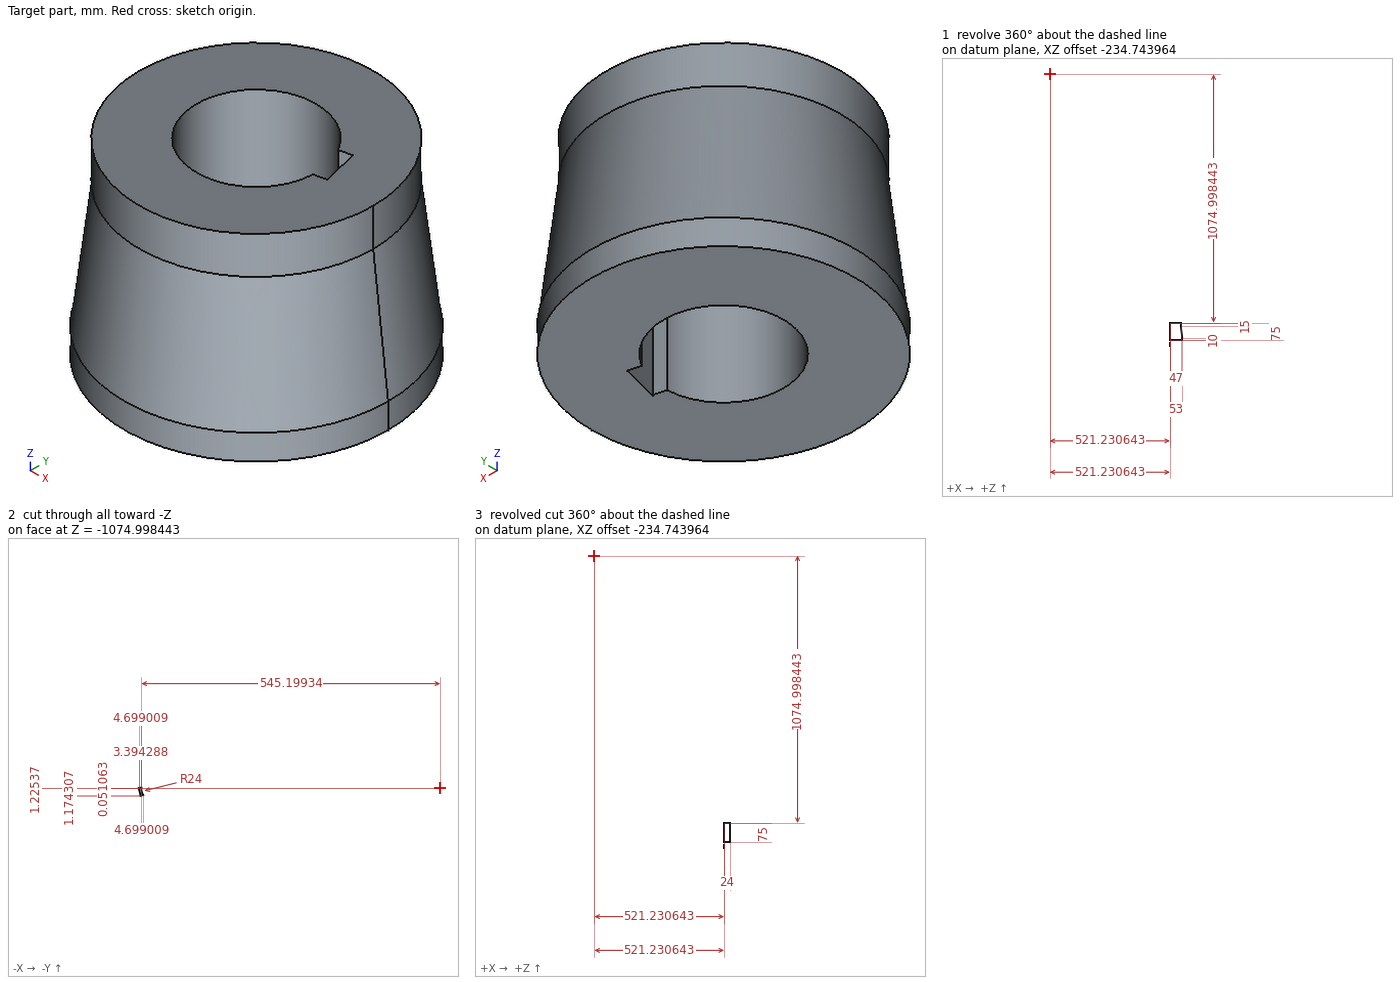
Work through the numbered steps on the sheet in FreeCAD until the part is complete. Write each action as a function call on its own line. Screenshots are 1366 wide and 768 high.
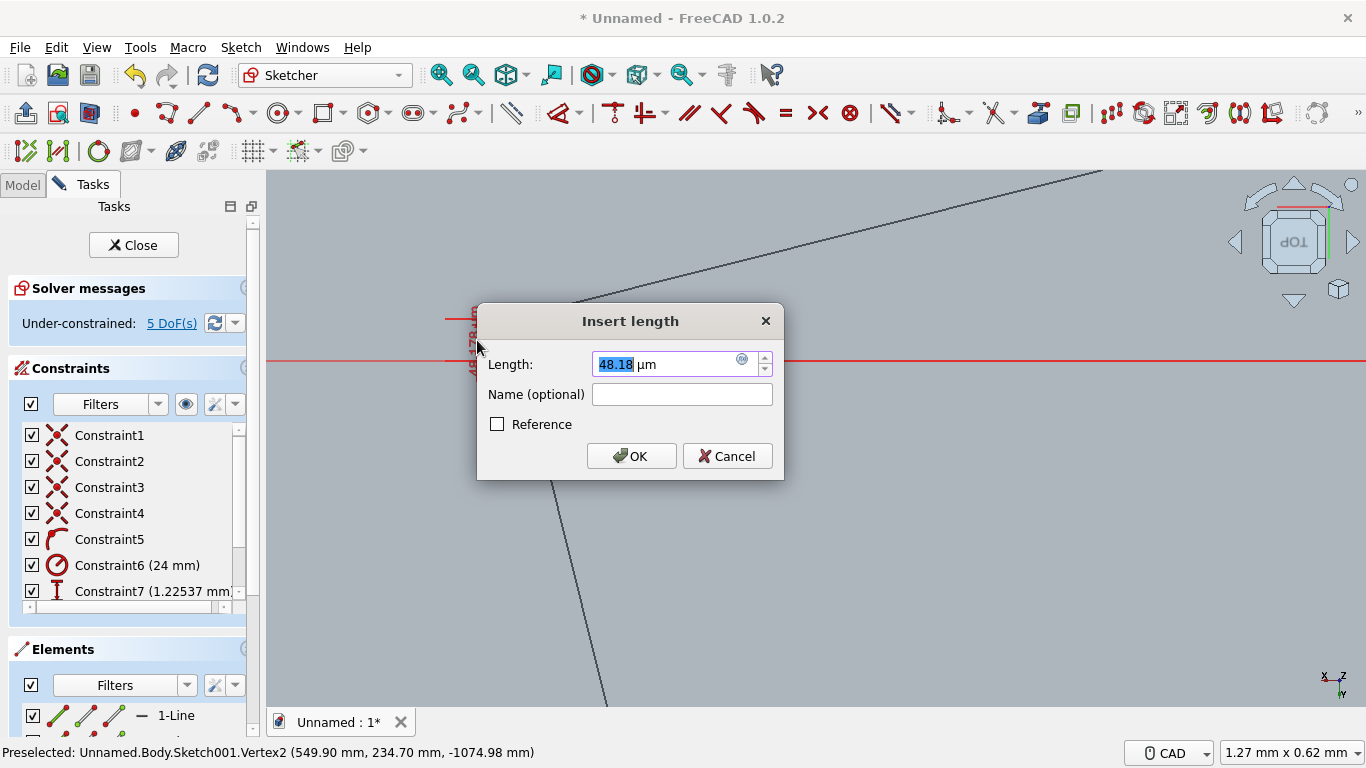
key(ctrl+a)
text(0.051063 mm)
key(Return)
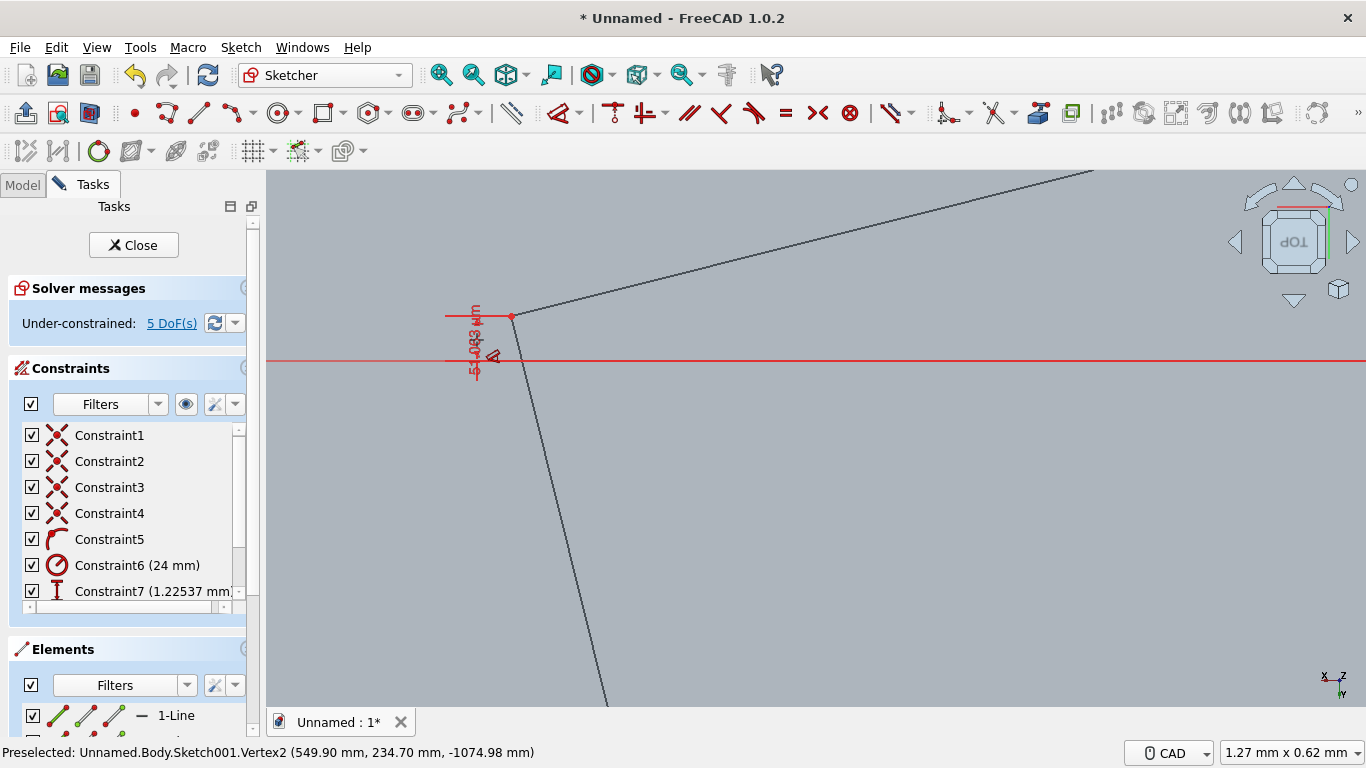
scroll(635, 257, down, 17)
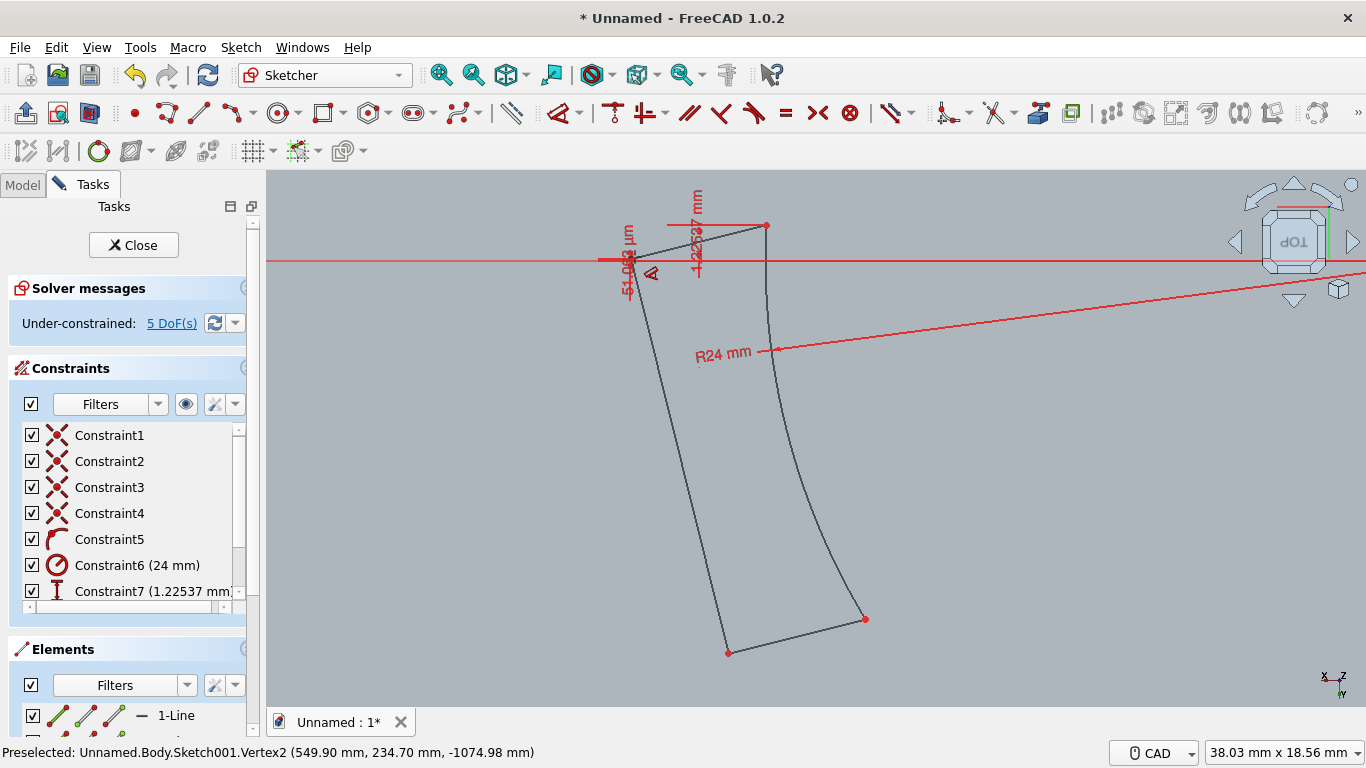
click(726, 235)
click(699, 293)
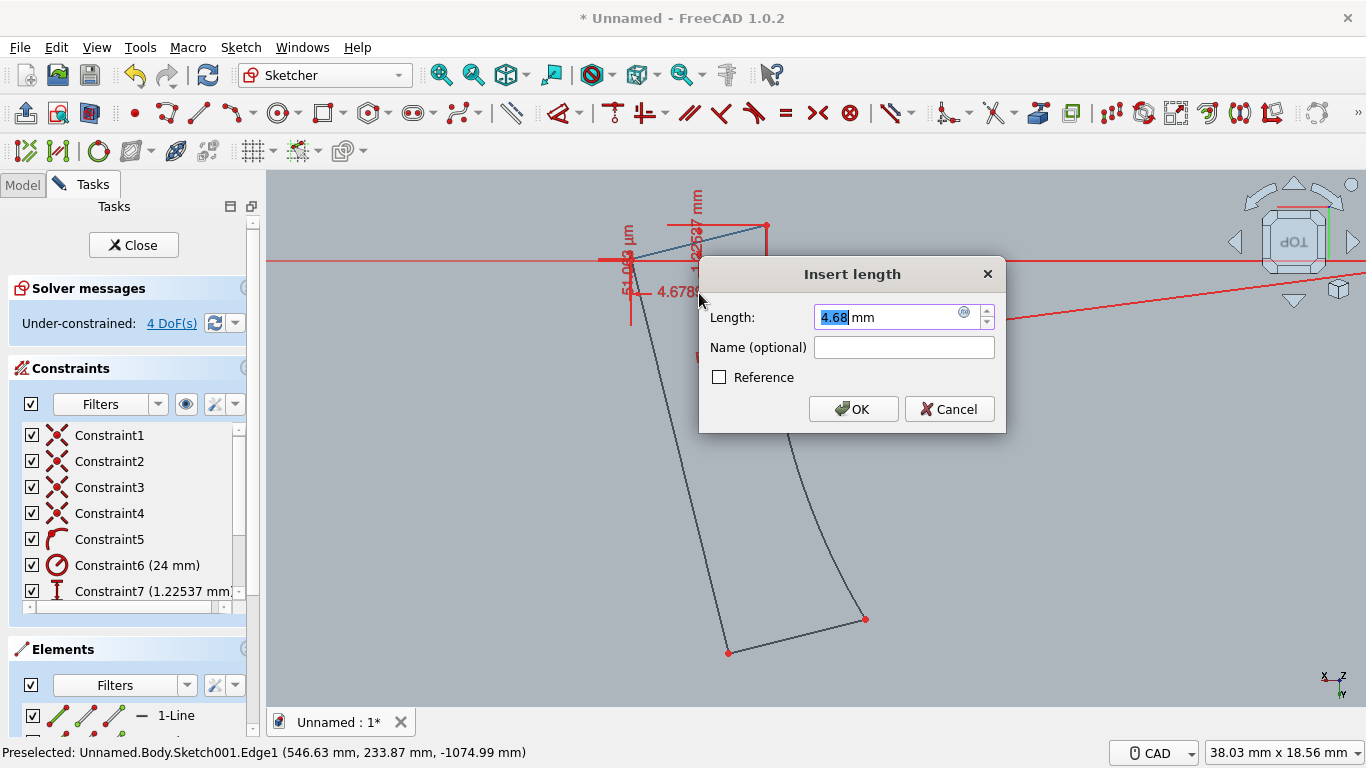
text(4.699009)
key(Return)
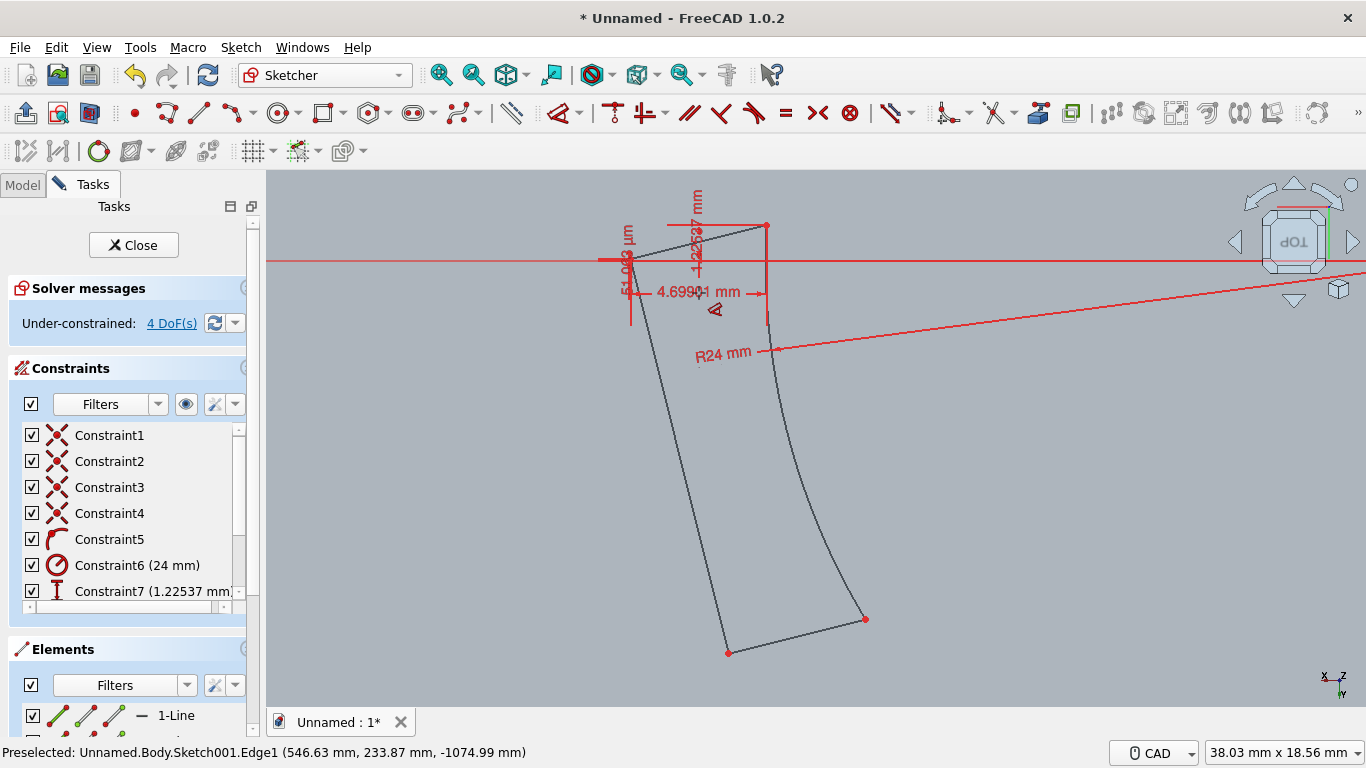
click(660, 378)
click(680, 201)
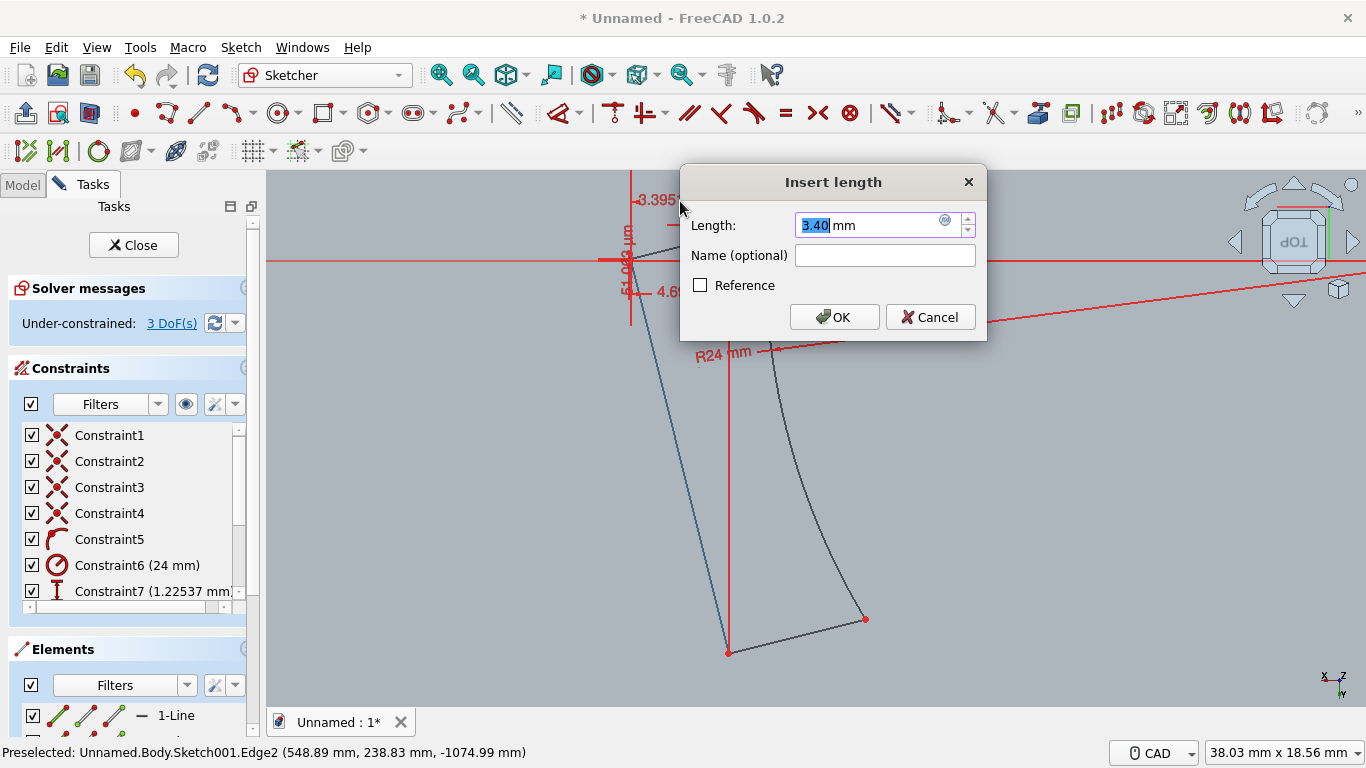
text(3.394288)
key(Return)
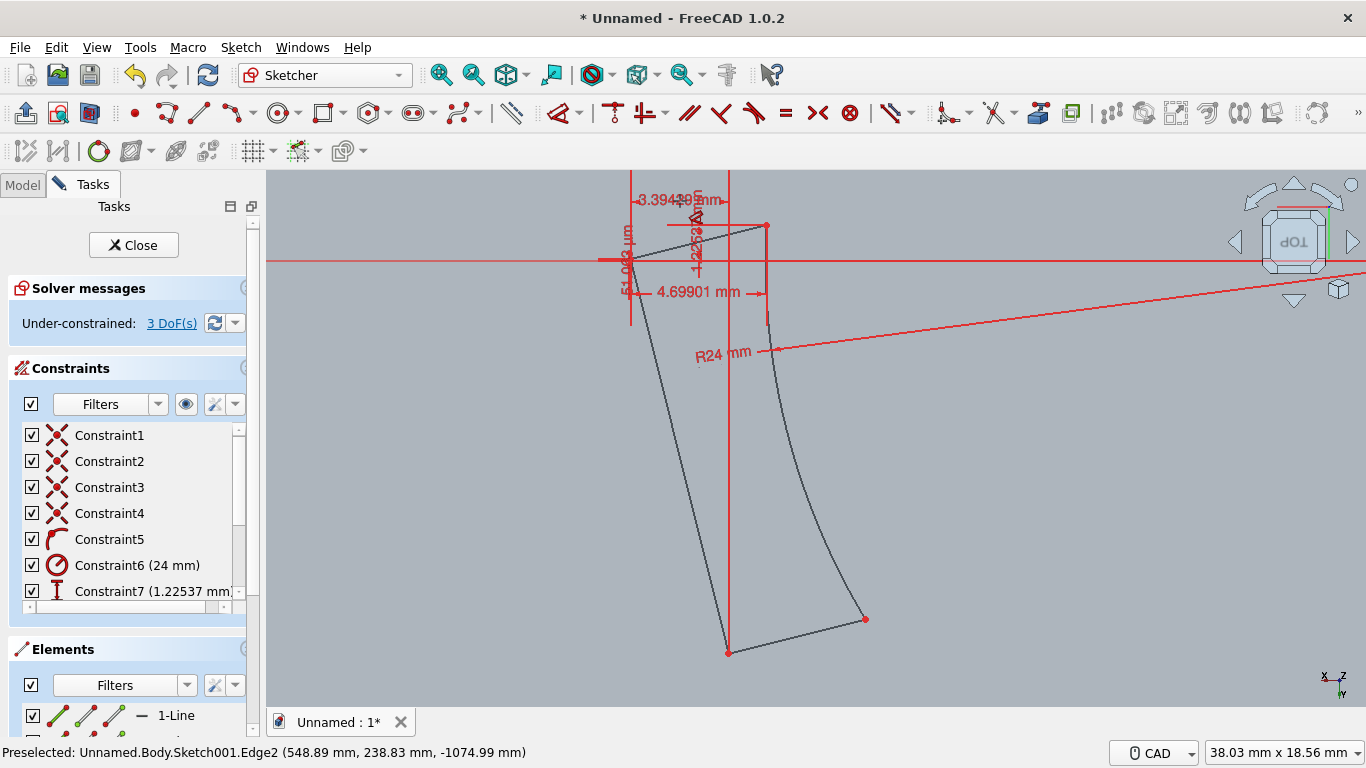
click(770, 643)
click(797, 586)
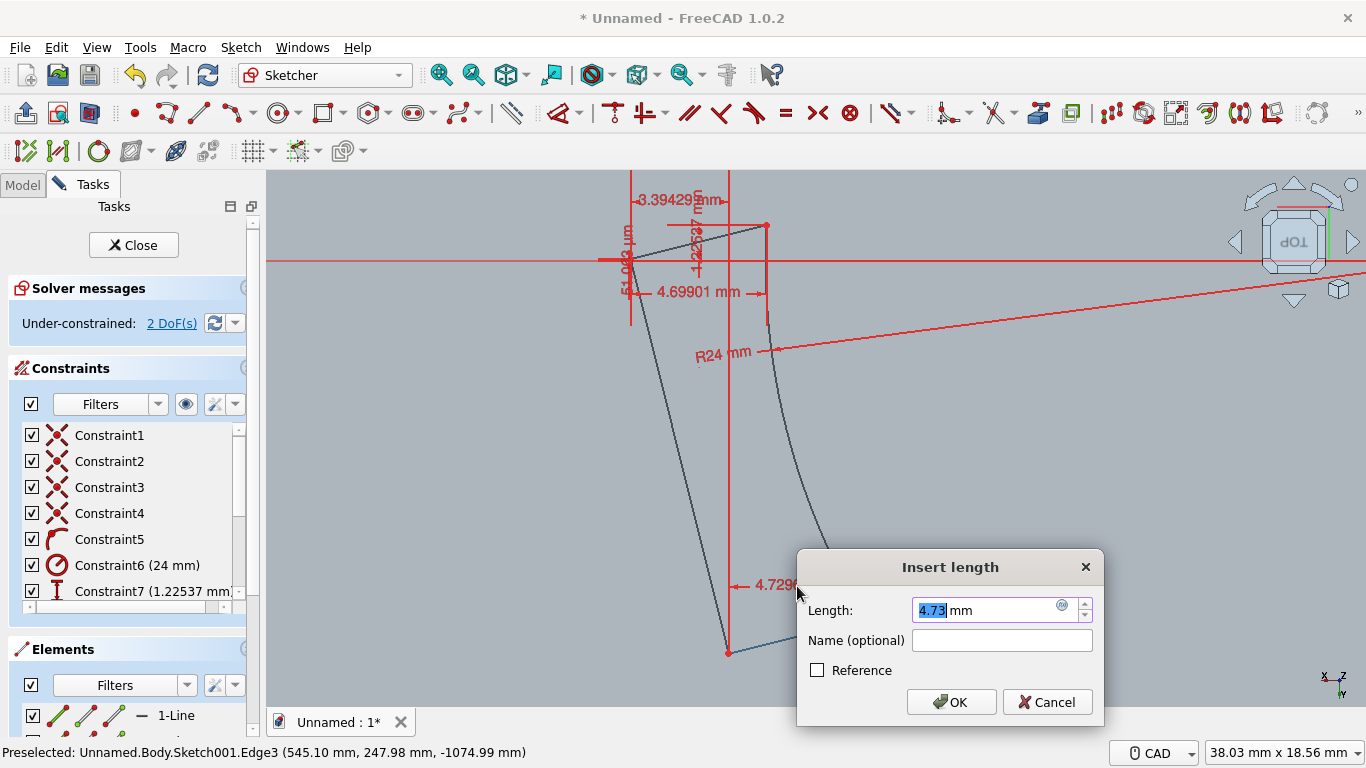
text(4.699009)
key(Return)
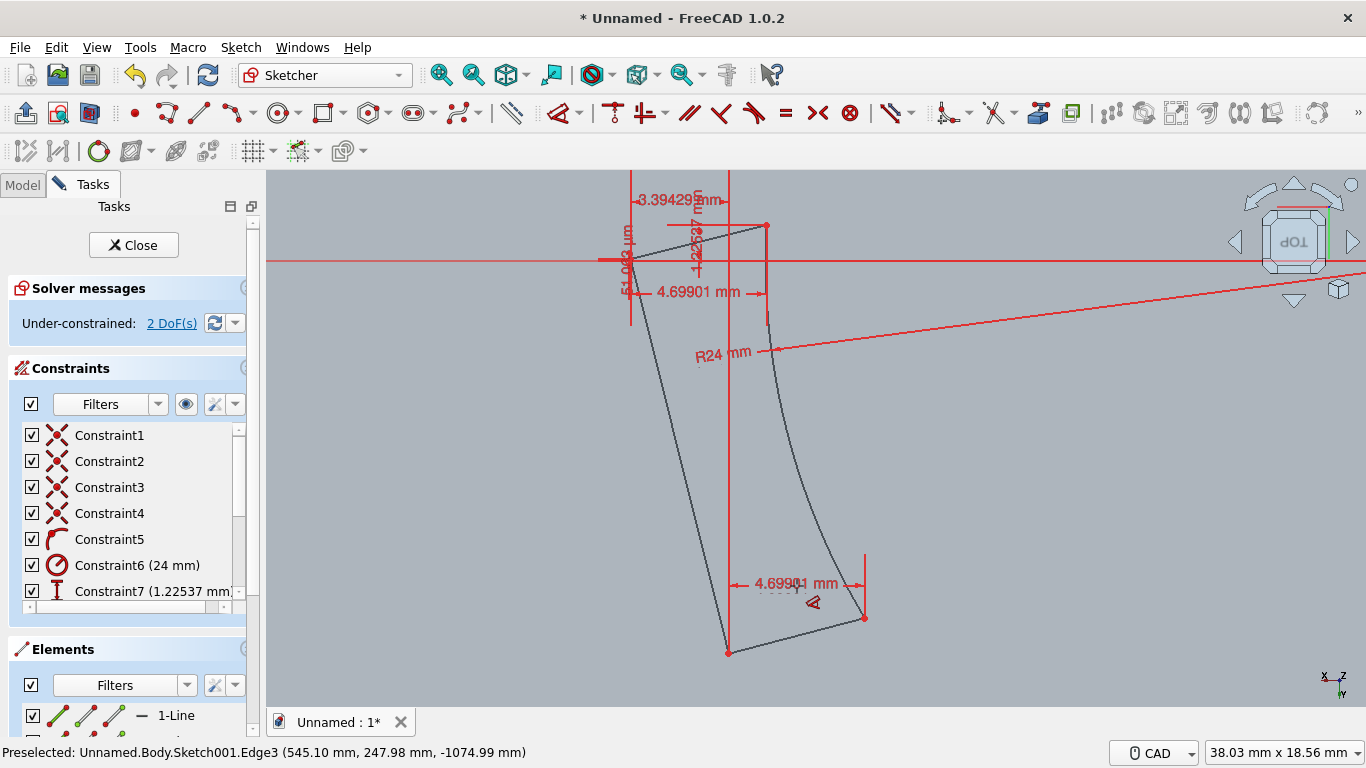
click(770, 643)
click(899, 636)